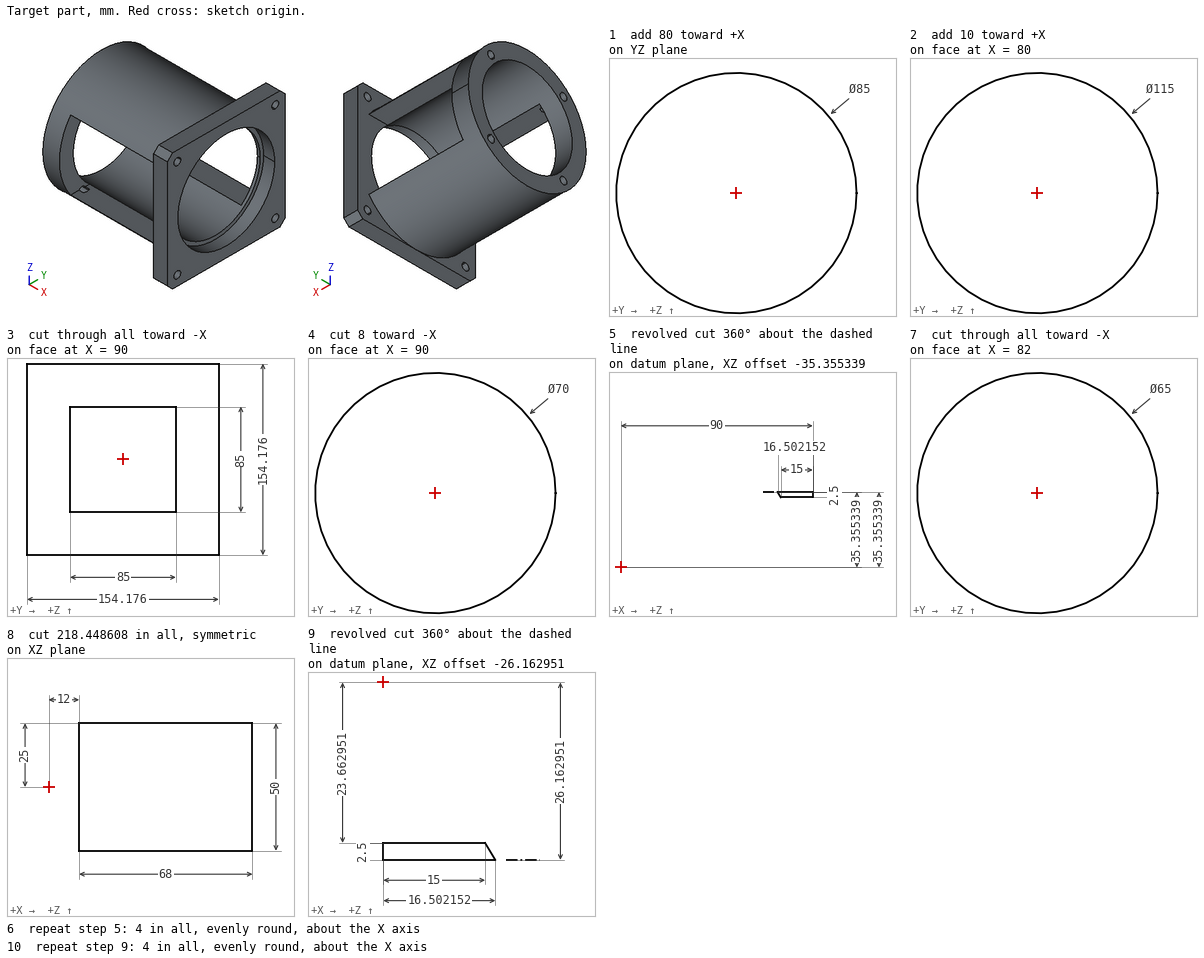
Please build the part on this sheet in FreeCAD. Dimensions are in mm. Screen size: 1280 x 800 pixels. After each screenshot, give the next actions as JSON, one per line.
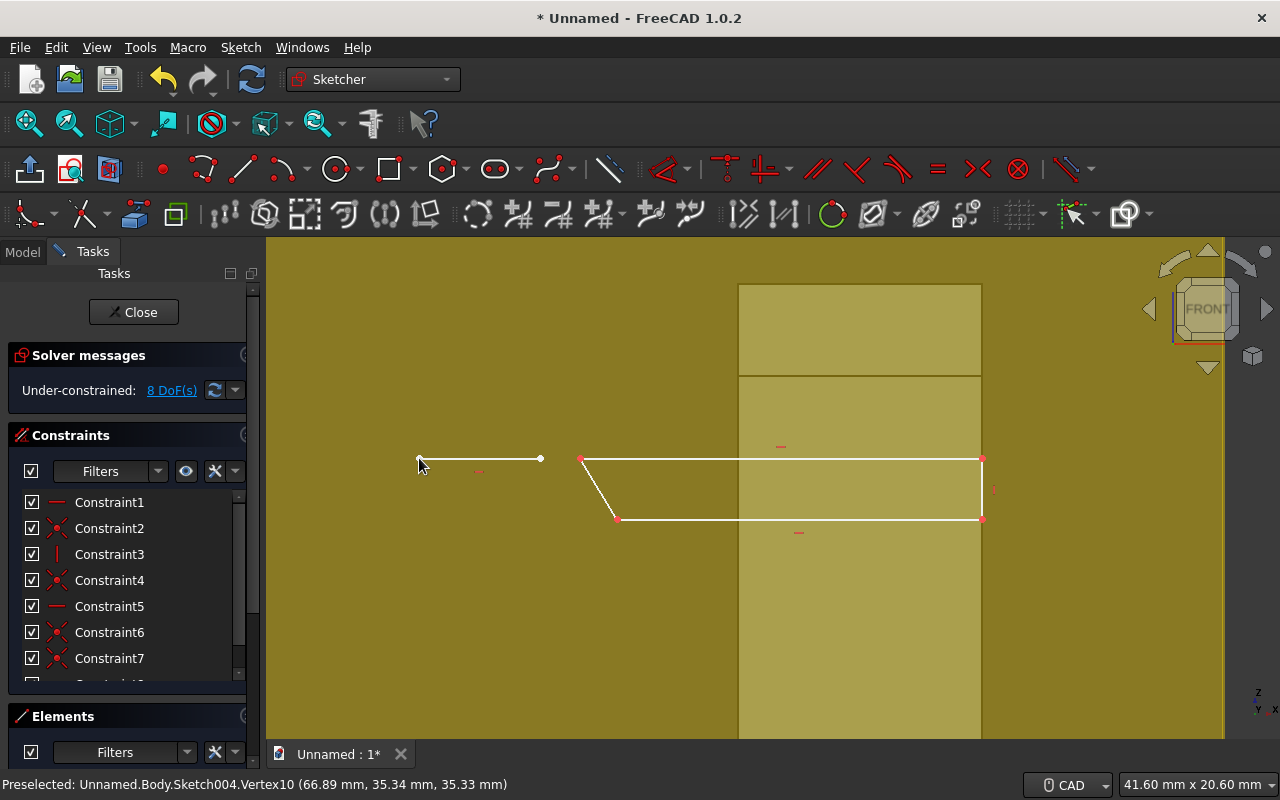
{"action": "left_click", "coordinate": [504, 459]}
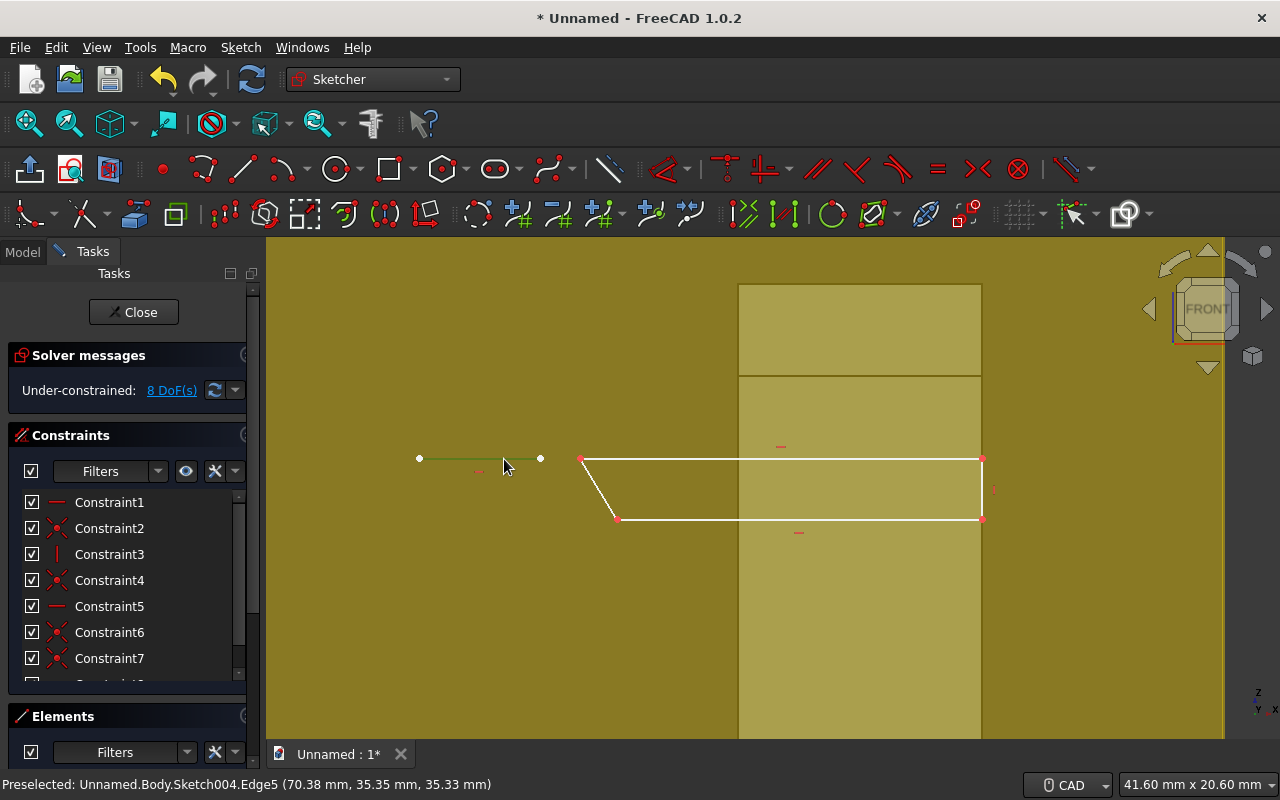
{"action": "key", "text": "g n"}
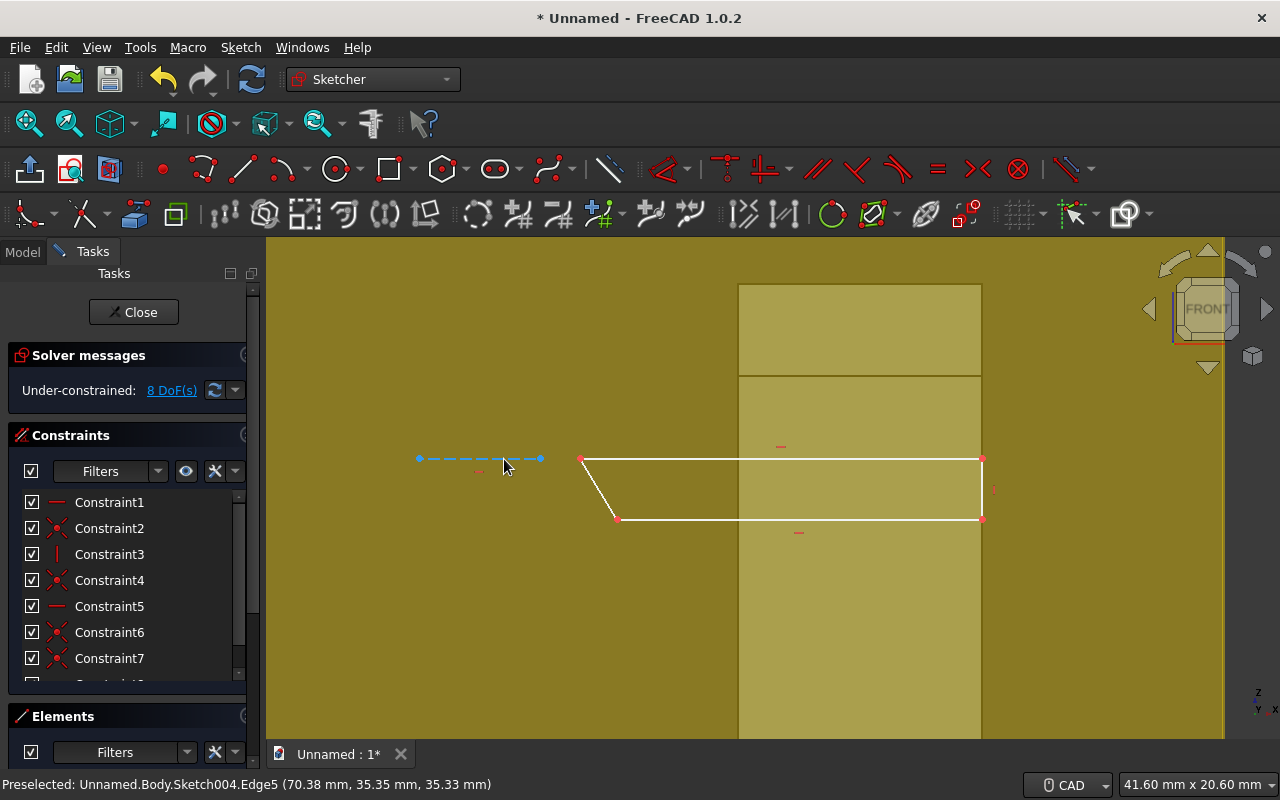
{"action": "left_click", "coordinate": [664, 170]}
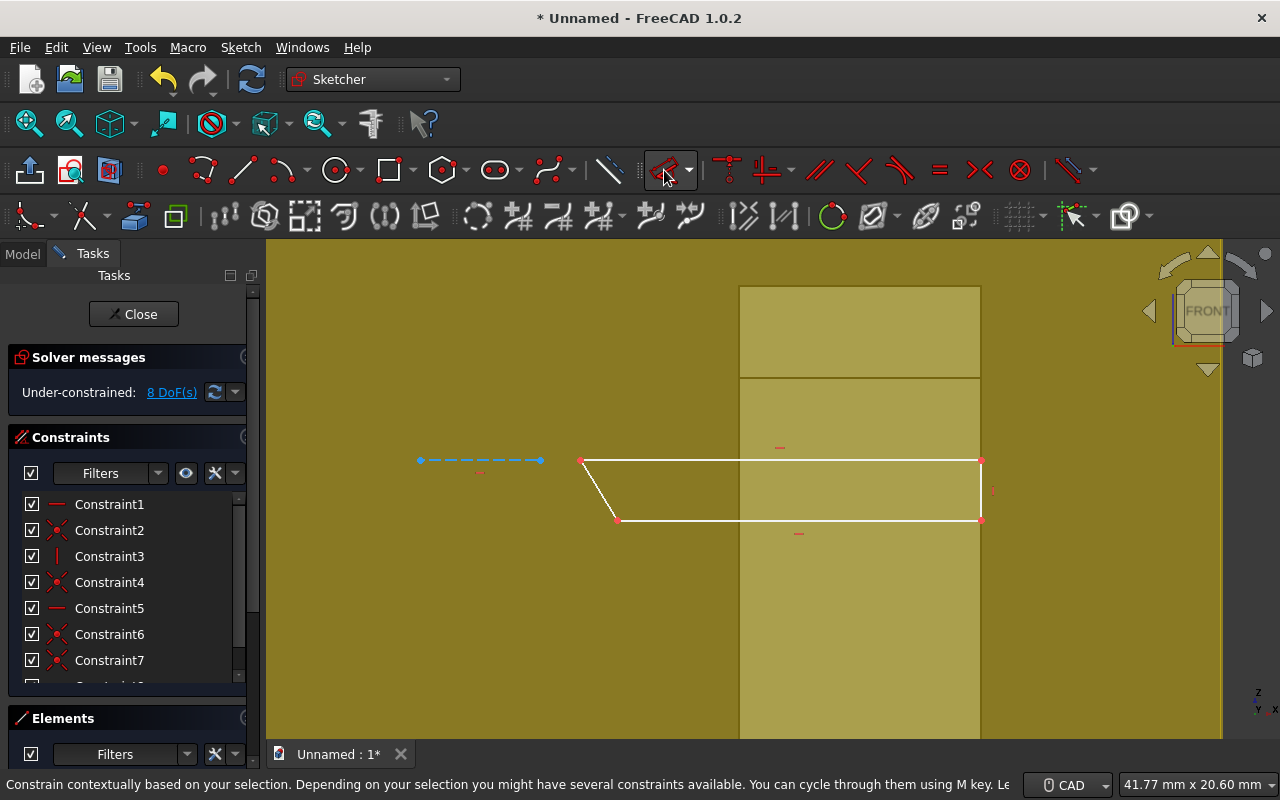
{"action": "left_click", "coordinate": [872, 521]}
{"action": "left_click", "coordinate": [799, 555]}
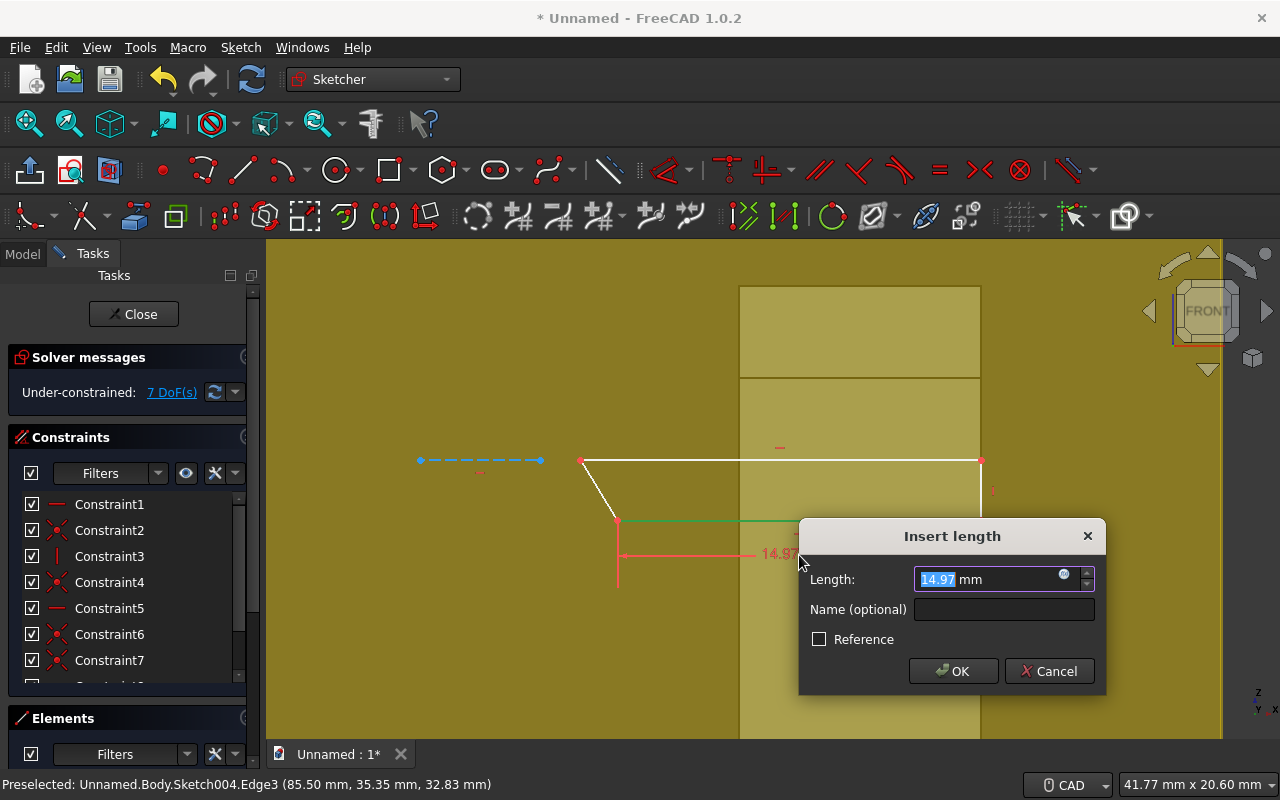
{"action": "type", "text": "15"}
{"action": "key", "text": "Return"}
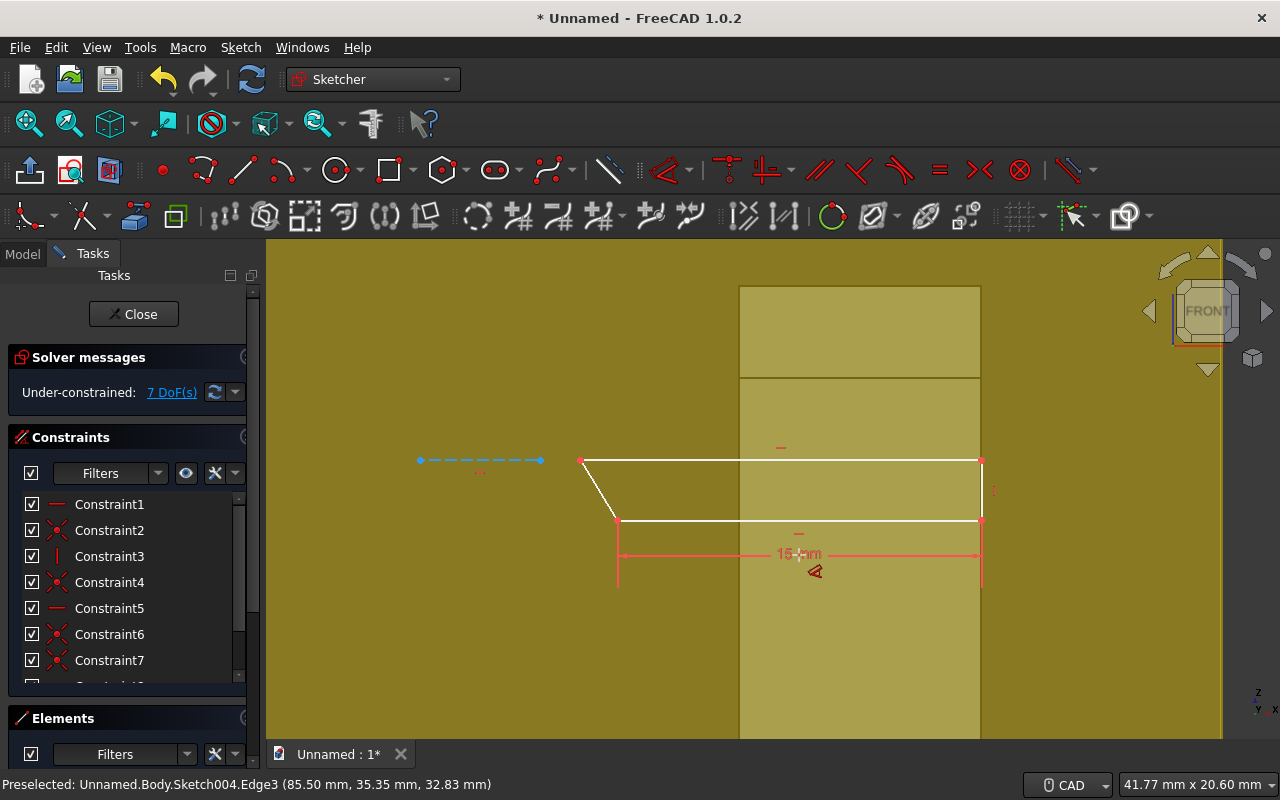
{"action": "left_click", "coordinate": [982, 478]}
{"action": "left_click", "coordinate": [1016, 490]}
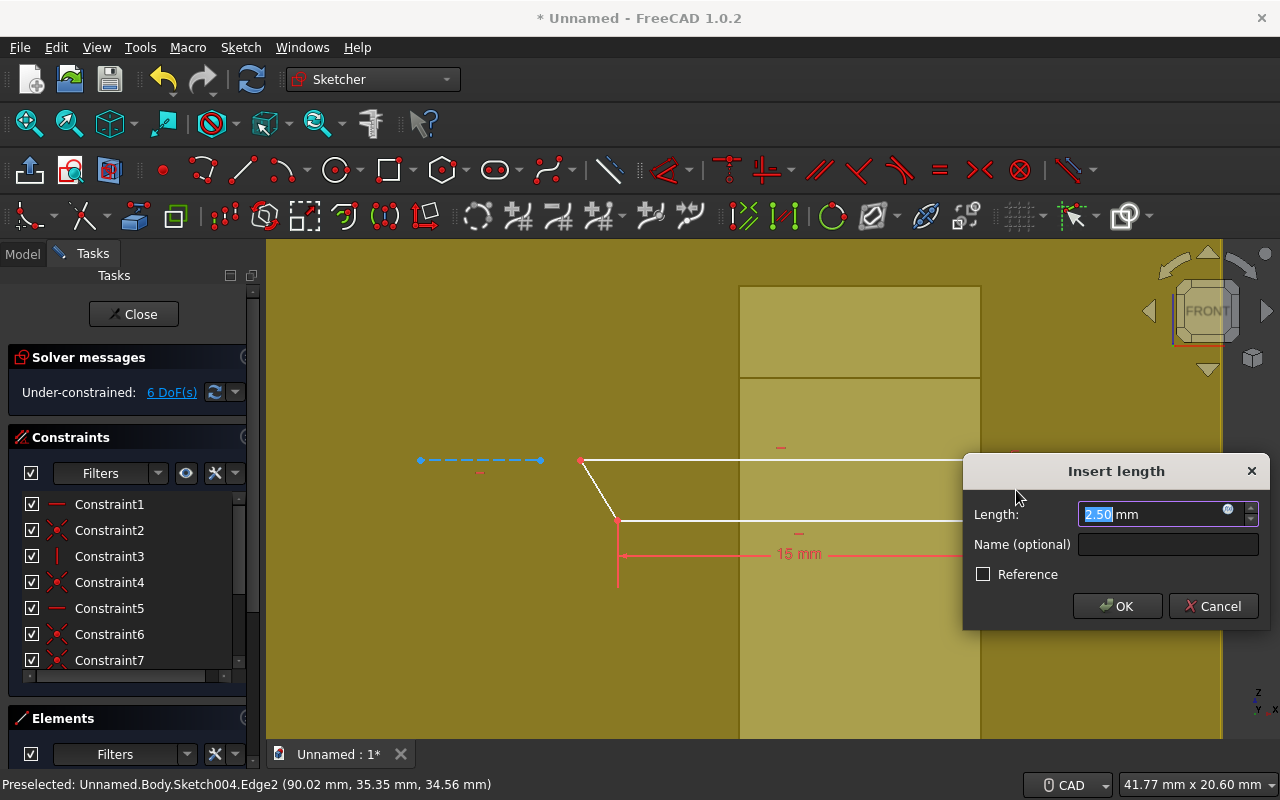
{"action": "type", "text": "2.5"}
{"action": "key", "text": "Return"}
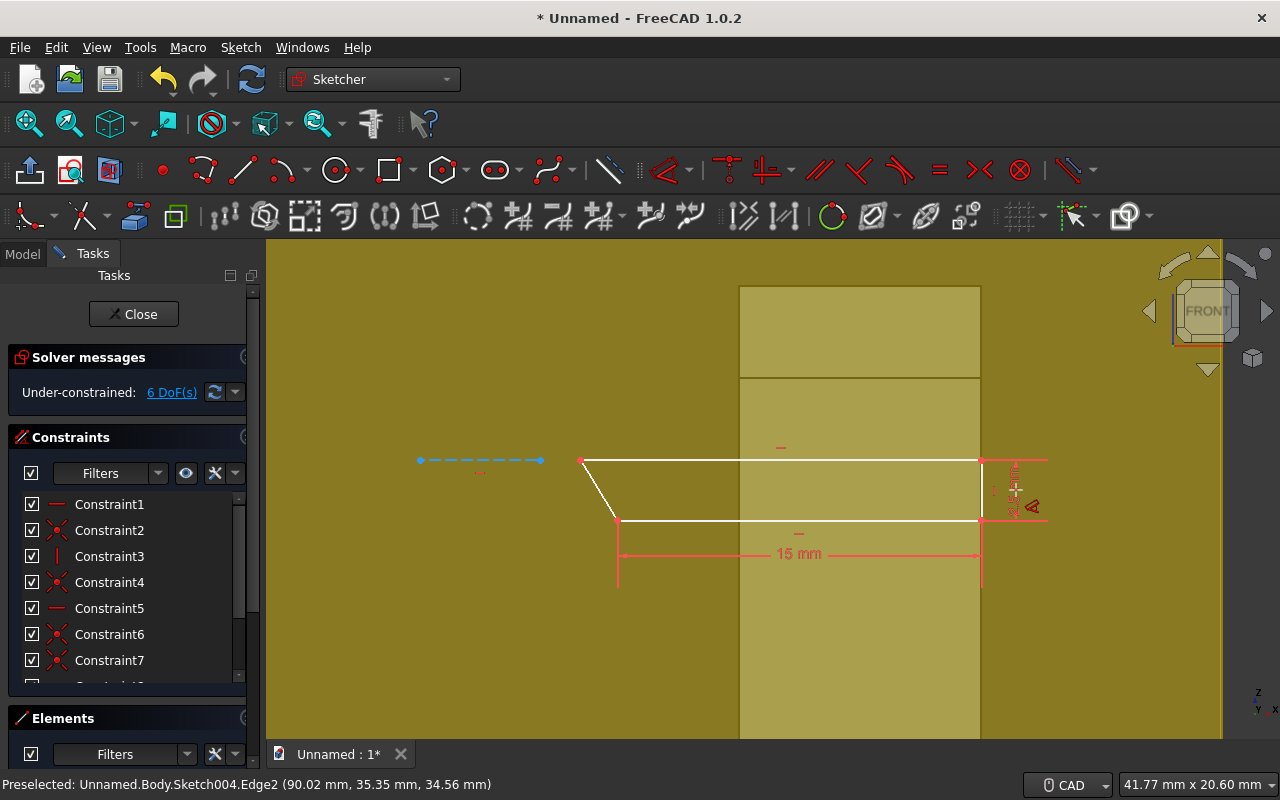
{"action": "left_click", "coordinate": [982, 460]}
{"action": "left_click", "coordinate": [638, 426]}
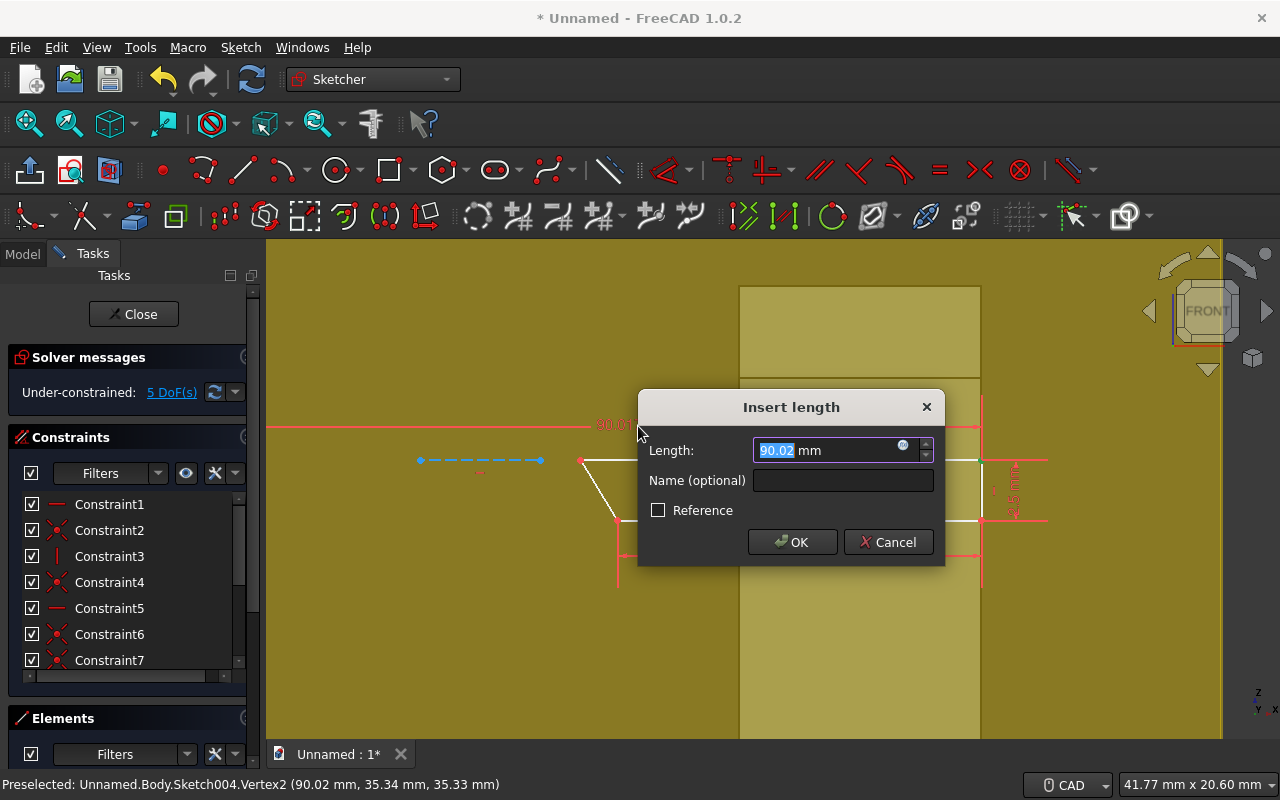
{"action": "type", "text": "90"}
{"action": "key", "text": "Return"}